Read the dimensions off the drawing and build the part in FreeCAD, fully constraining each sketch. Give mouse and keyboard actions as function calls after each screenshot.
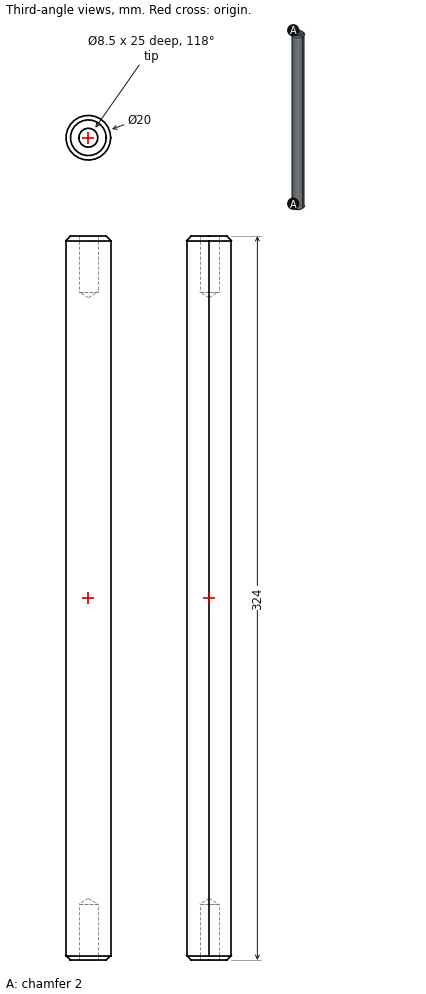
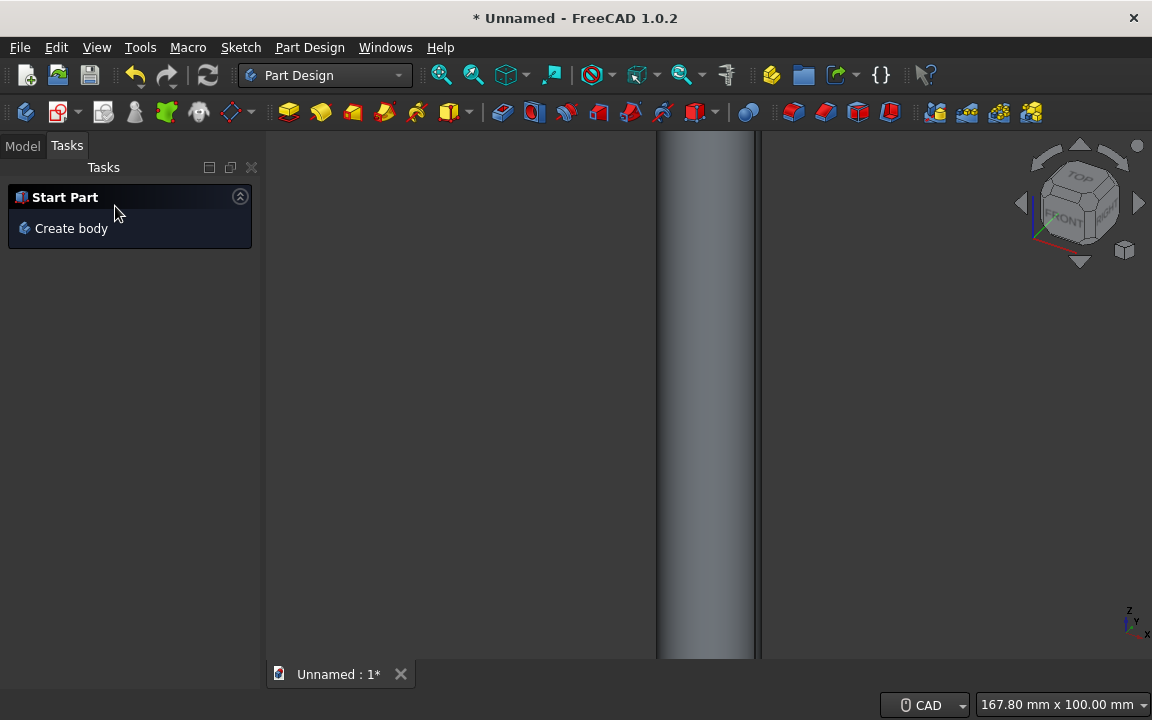
click(442, 76)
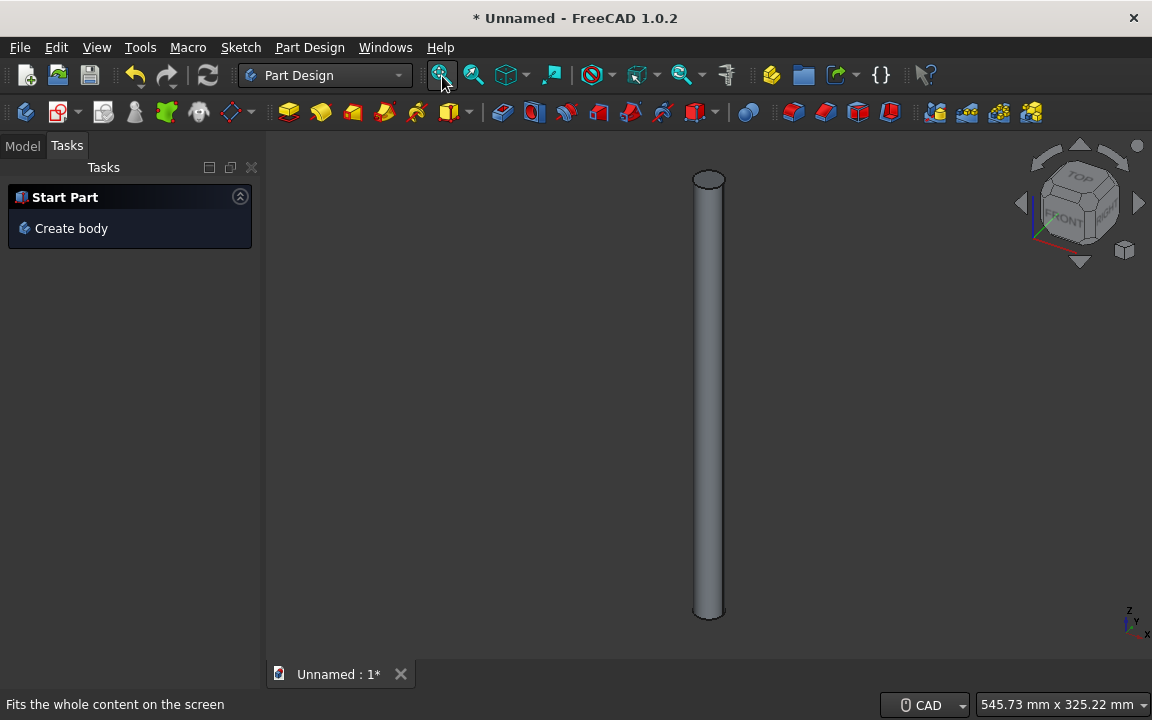
click(697, 616)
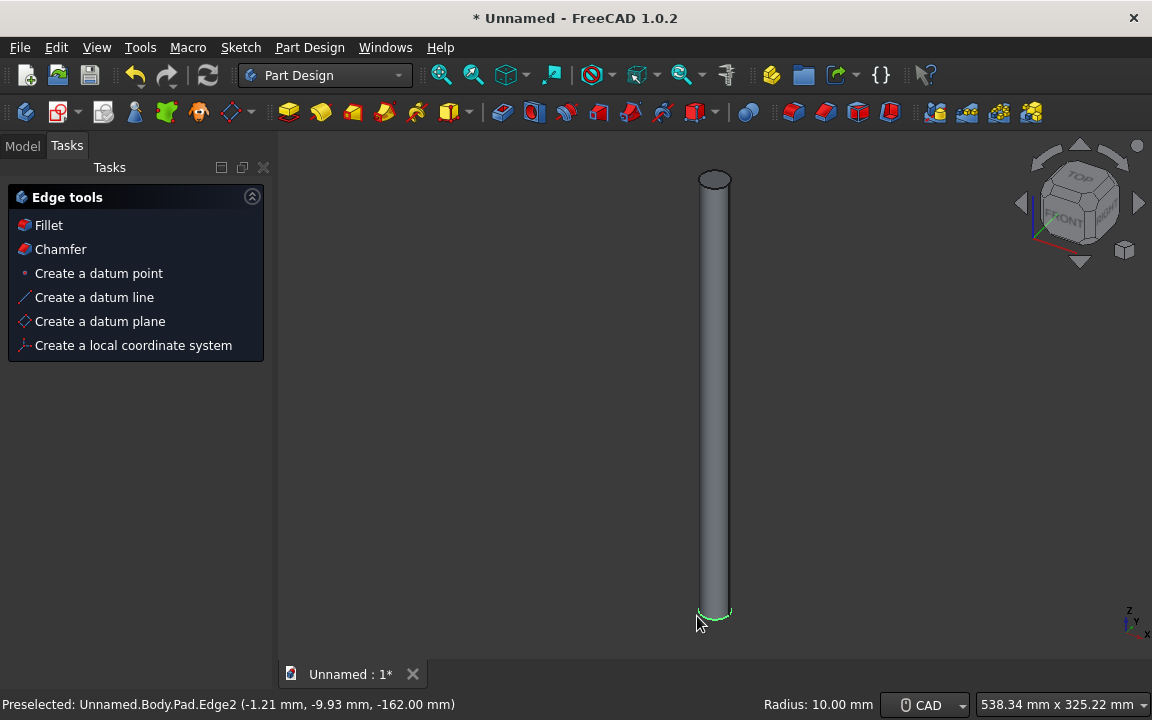
click(701, 174, ctrl)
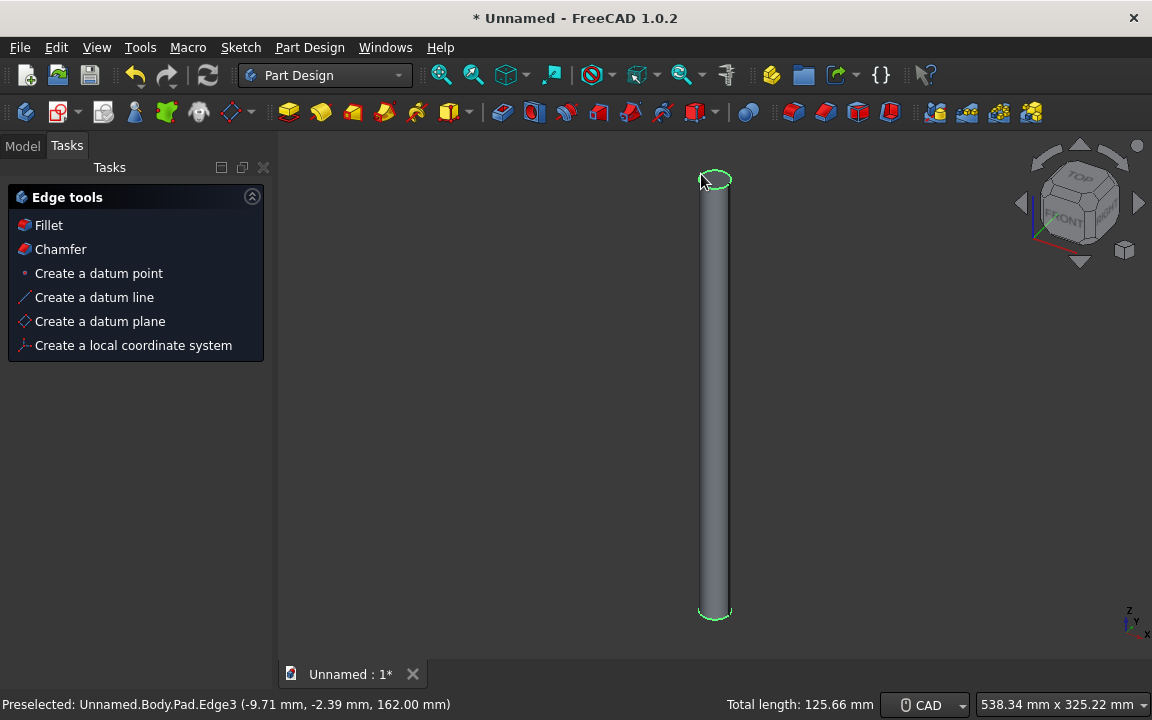
click(826, 112)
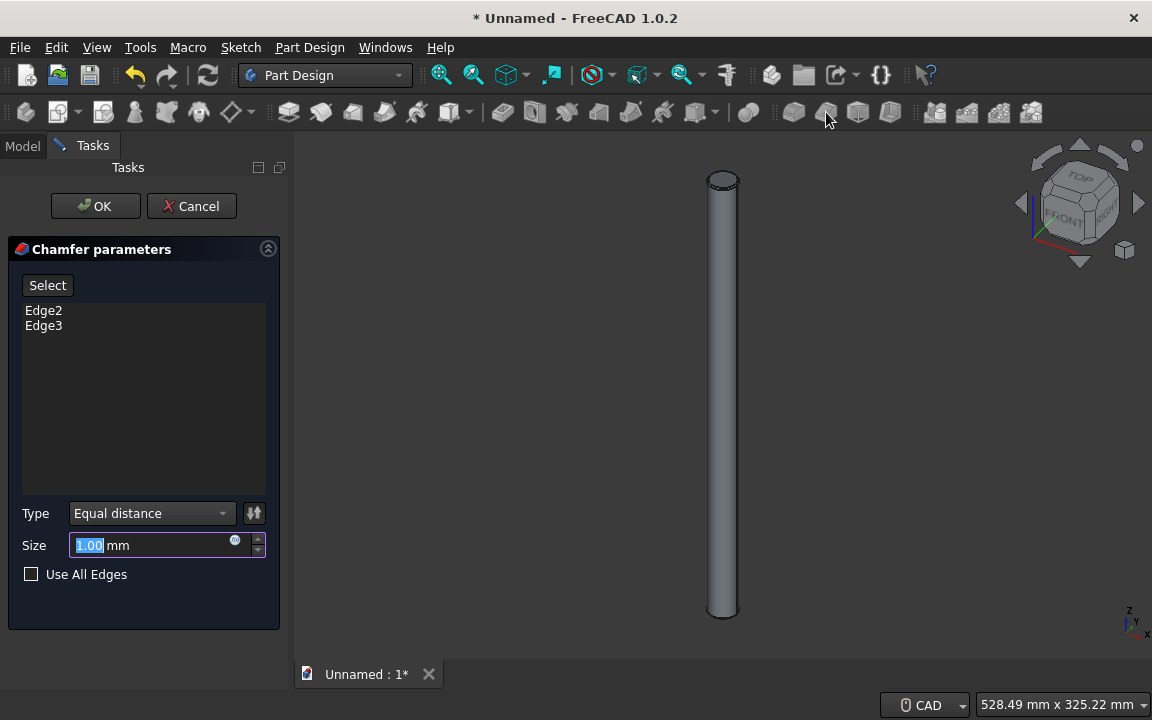
text(2)
key(Tab)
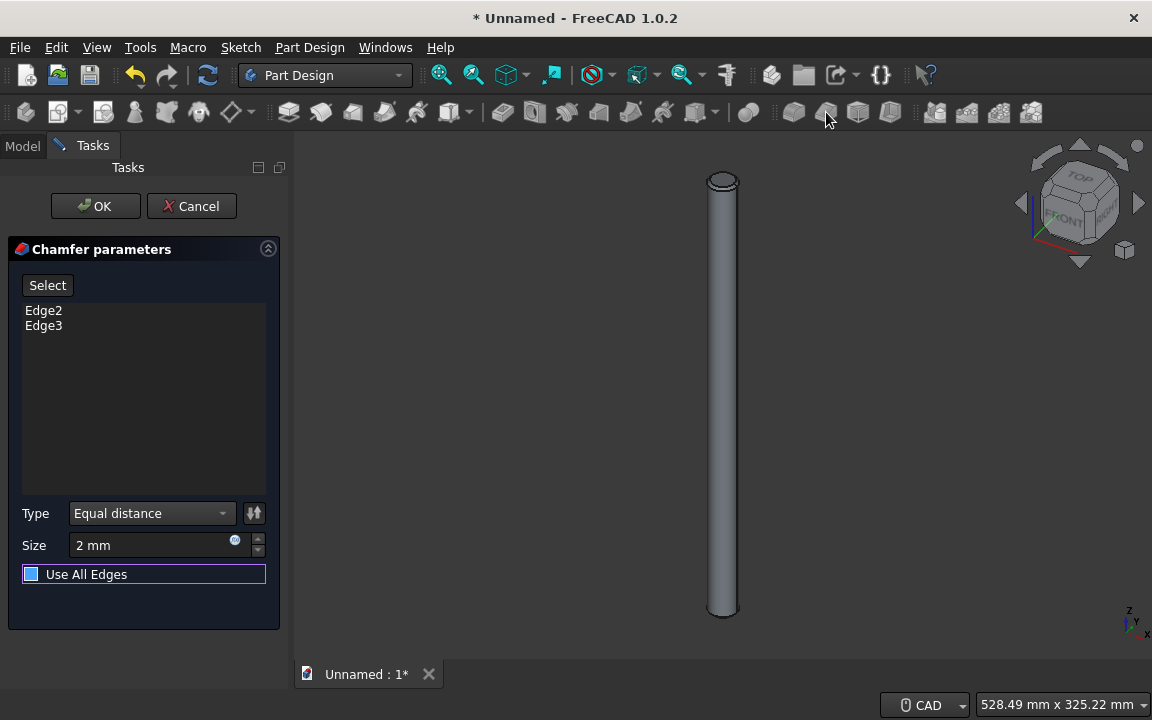
click(96, 206)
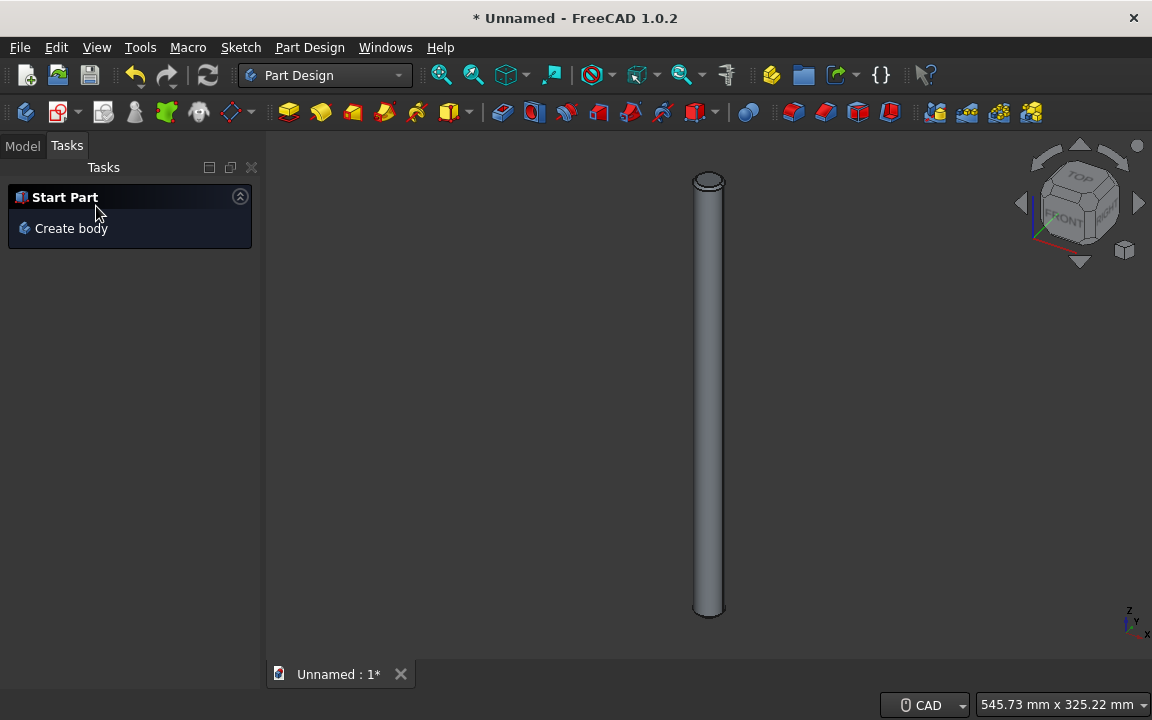
click(711, 177)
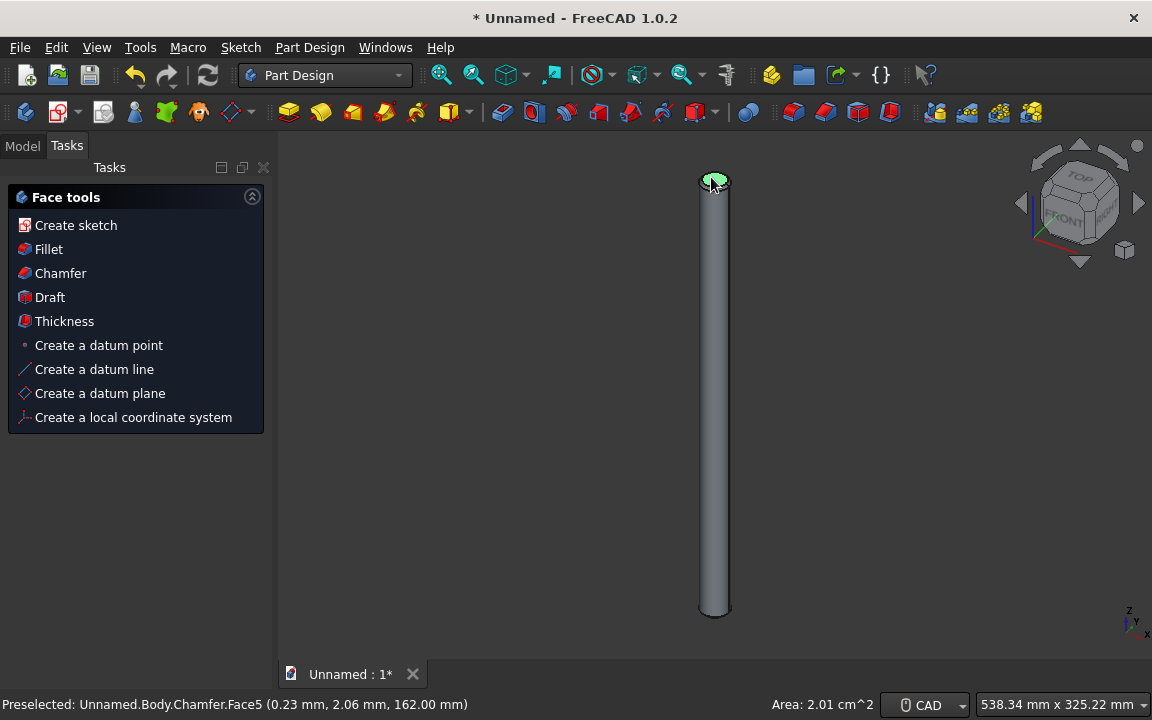
click(58, 112)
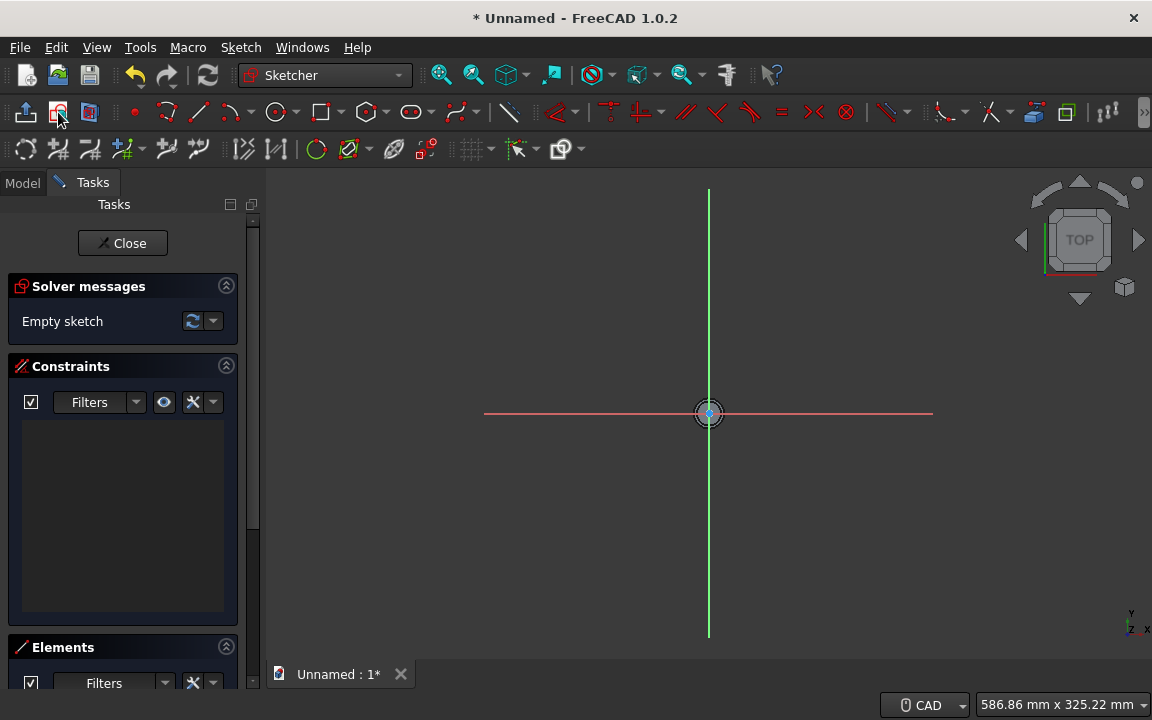
scroll(713, 414, up, 15)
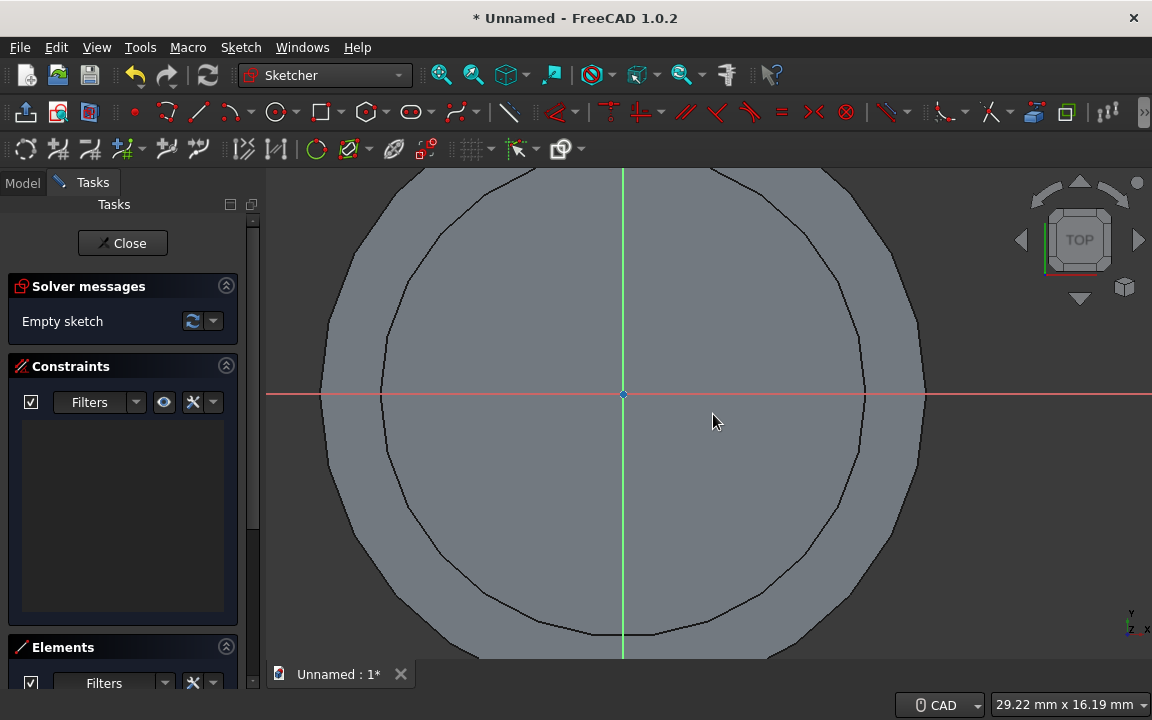
click(276, 112)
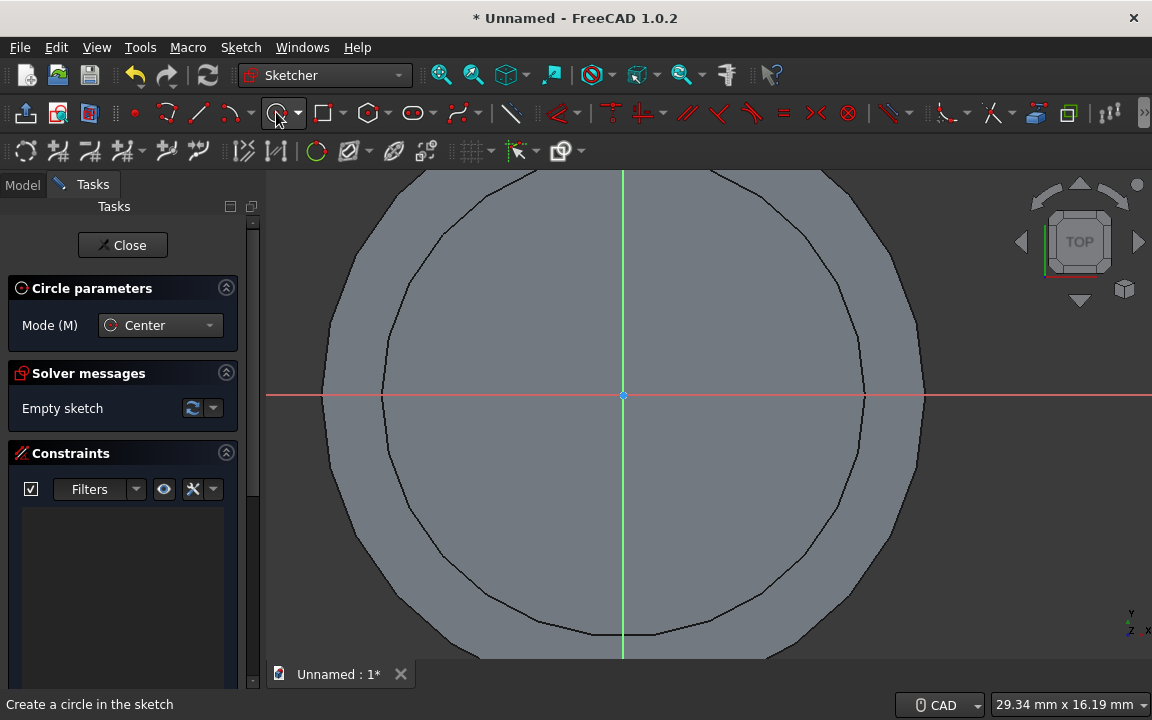
click(623, 395)
move(714, 305)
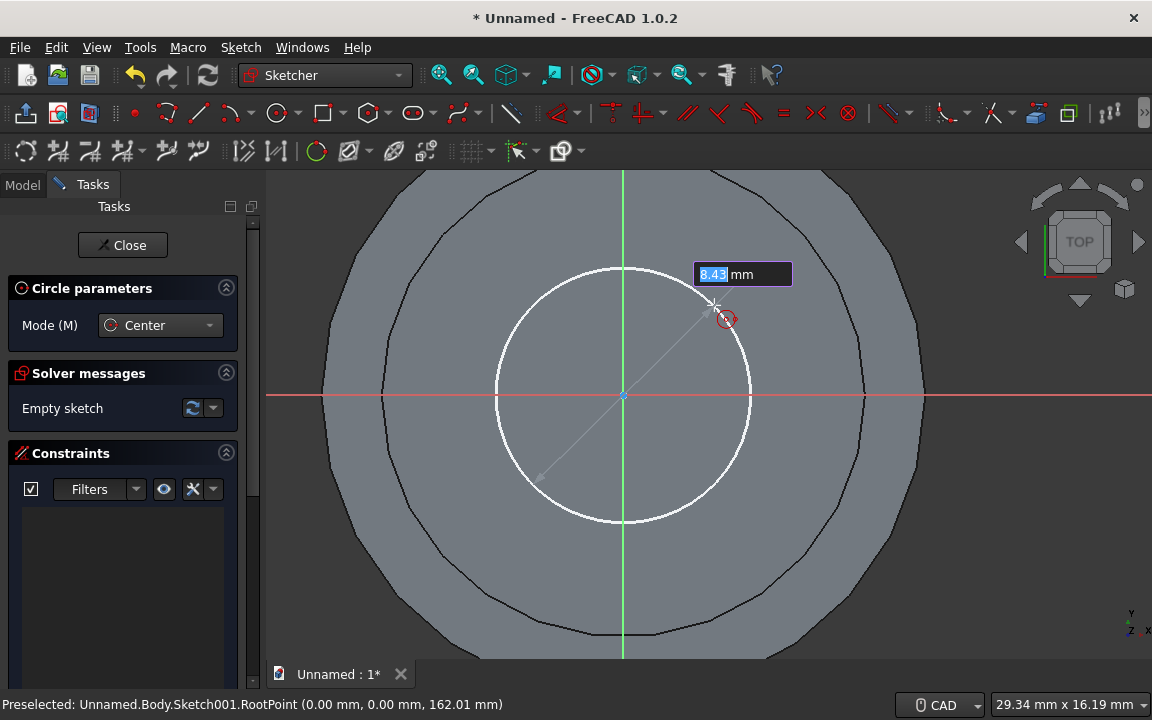
text(8.5)
key(Return)
key(Escape)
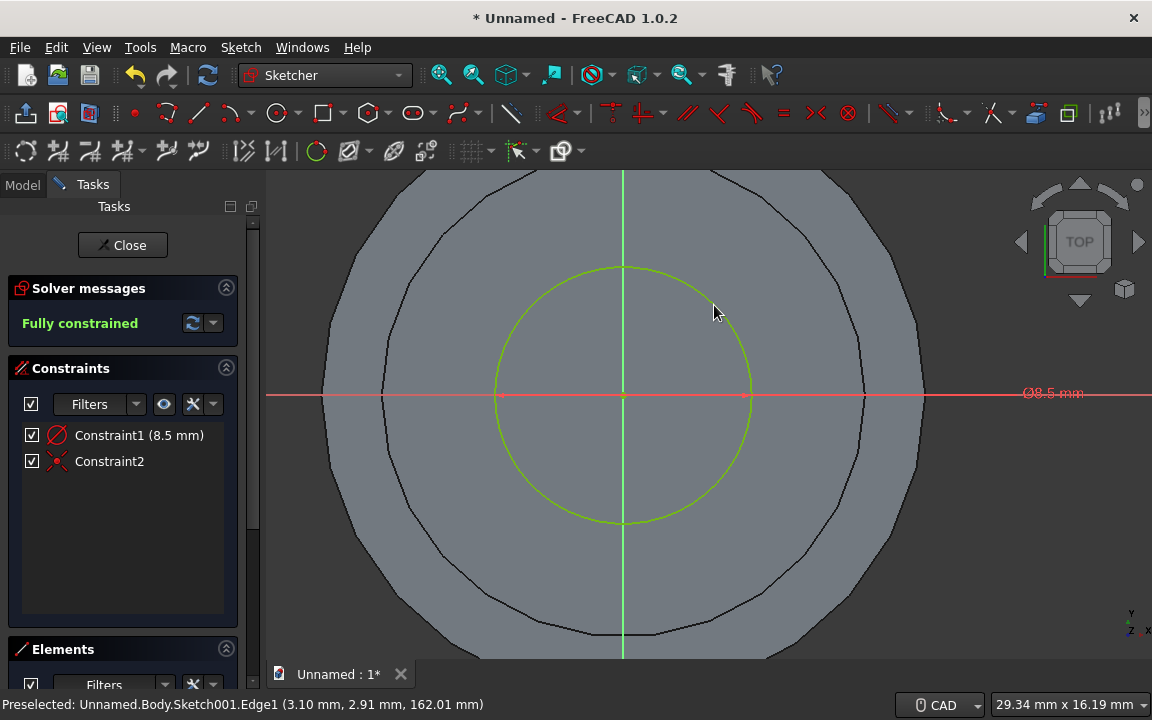
click(123, 245)